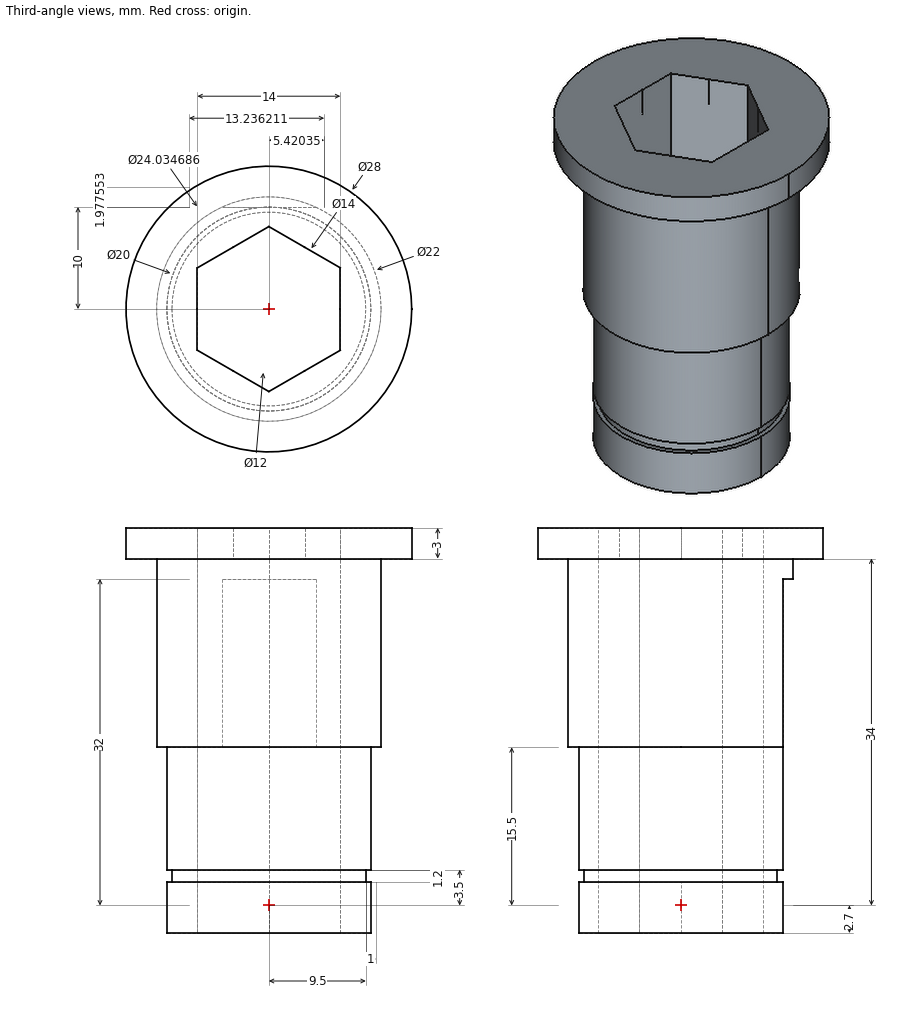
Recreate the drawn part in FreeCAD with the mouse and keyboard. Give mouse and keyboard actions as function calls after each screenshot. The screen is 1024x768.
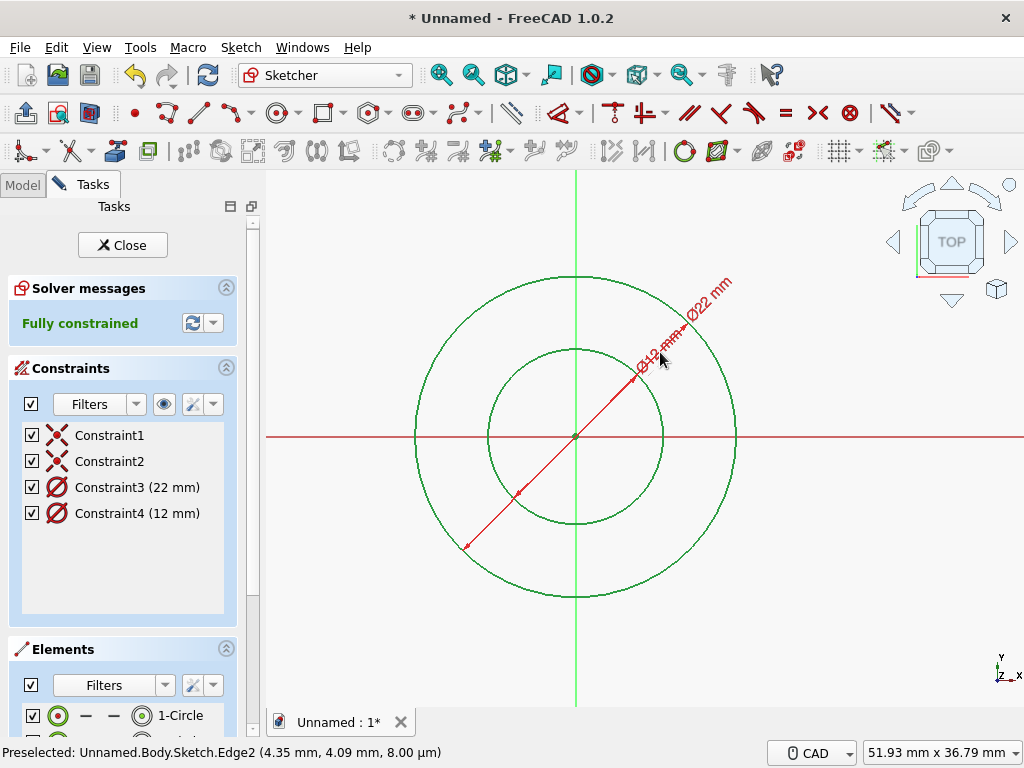
click(123, 245)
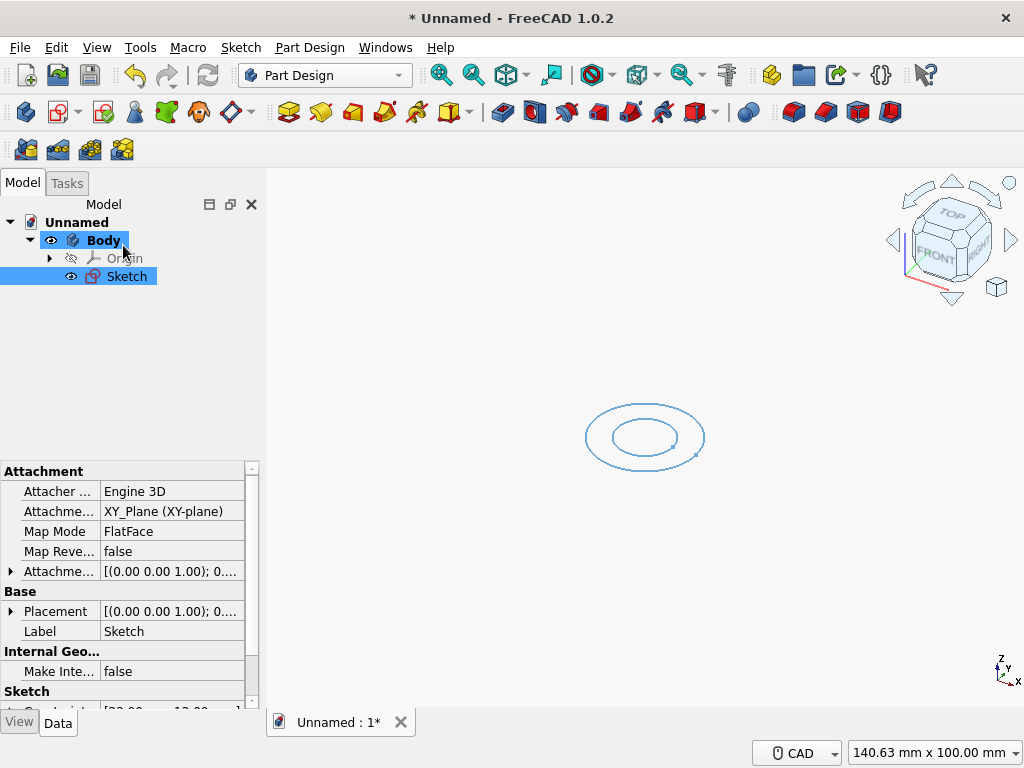
click(290, 112)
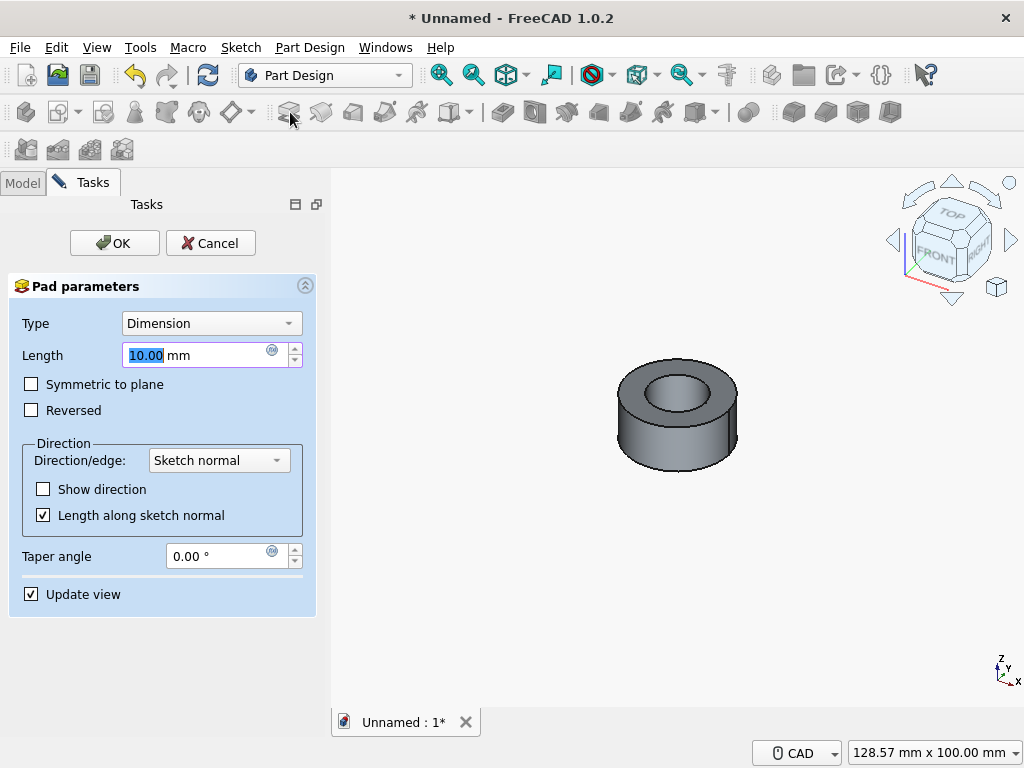
text(34)
key(Tab)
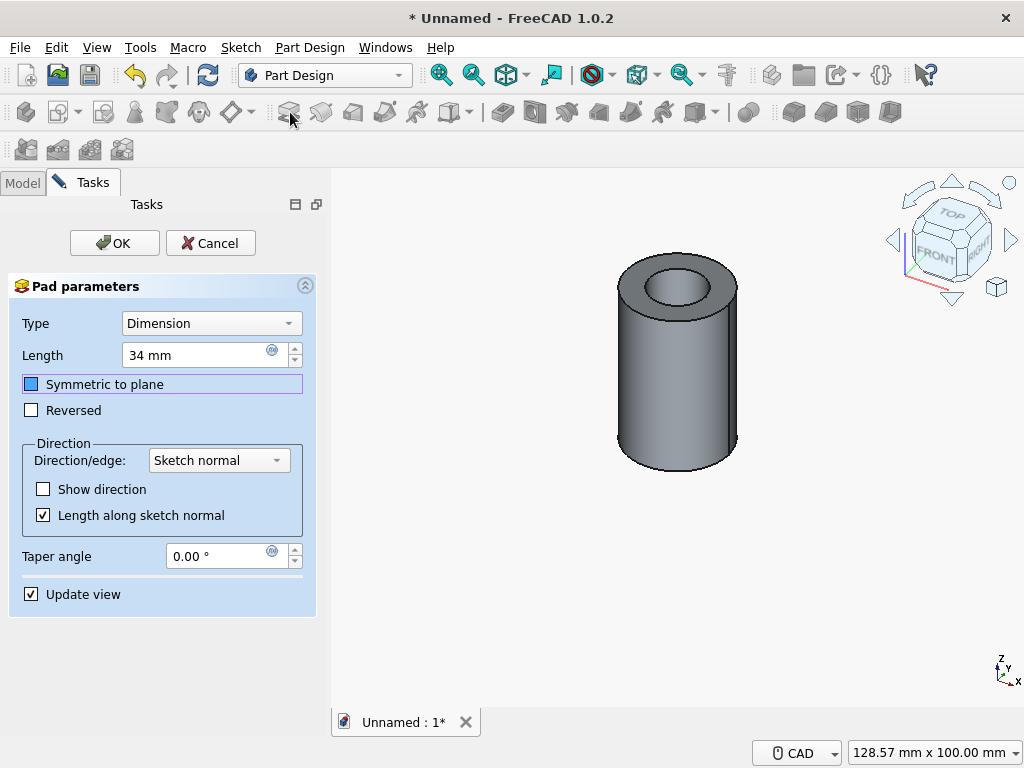
click(115, 243)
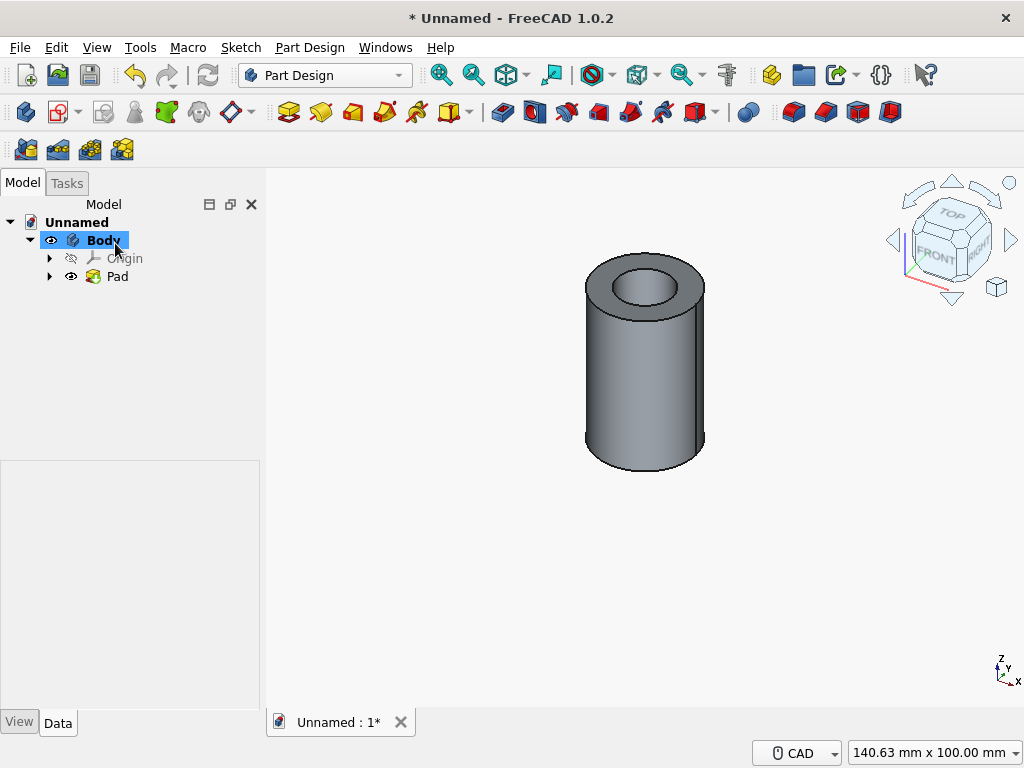
click(691, 279)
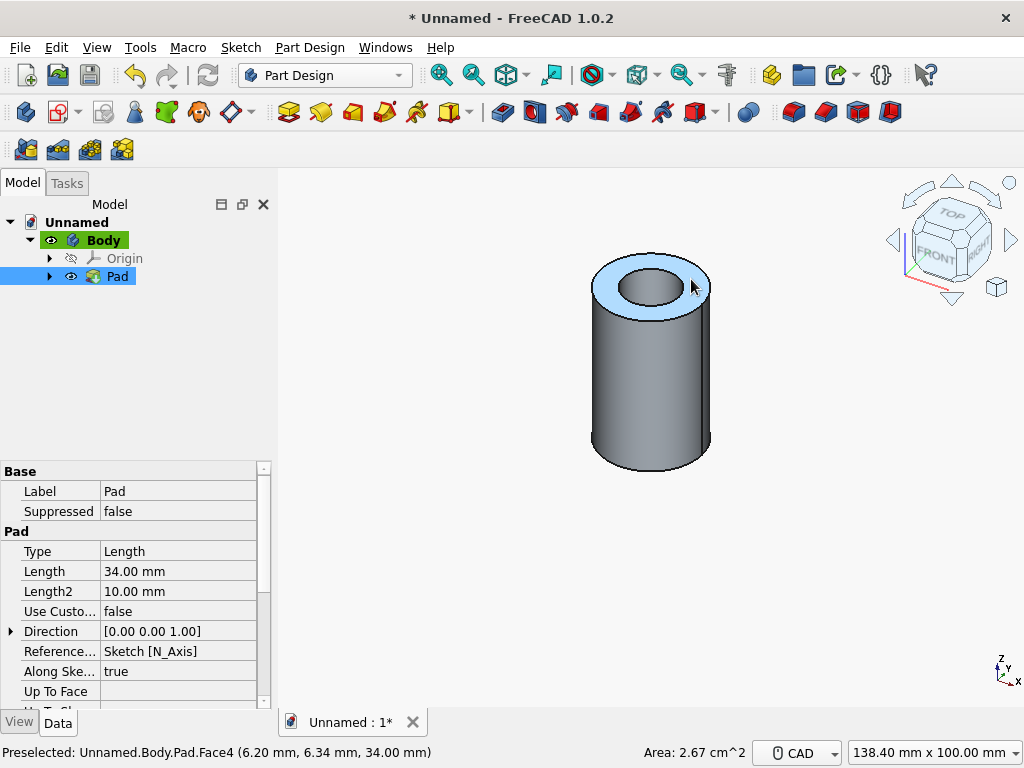
click(58, 112)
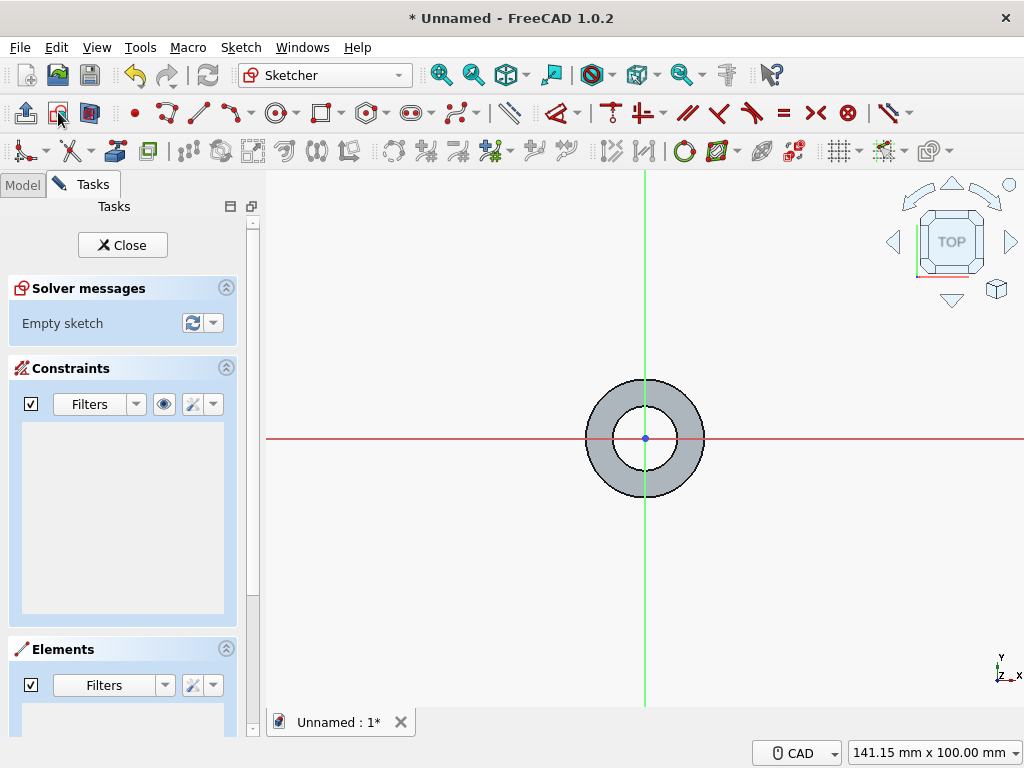
scroll(701, 438, up, 4)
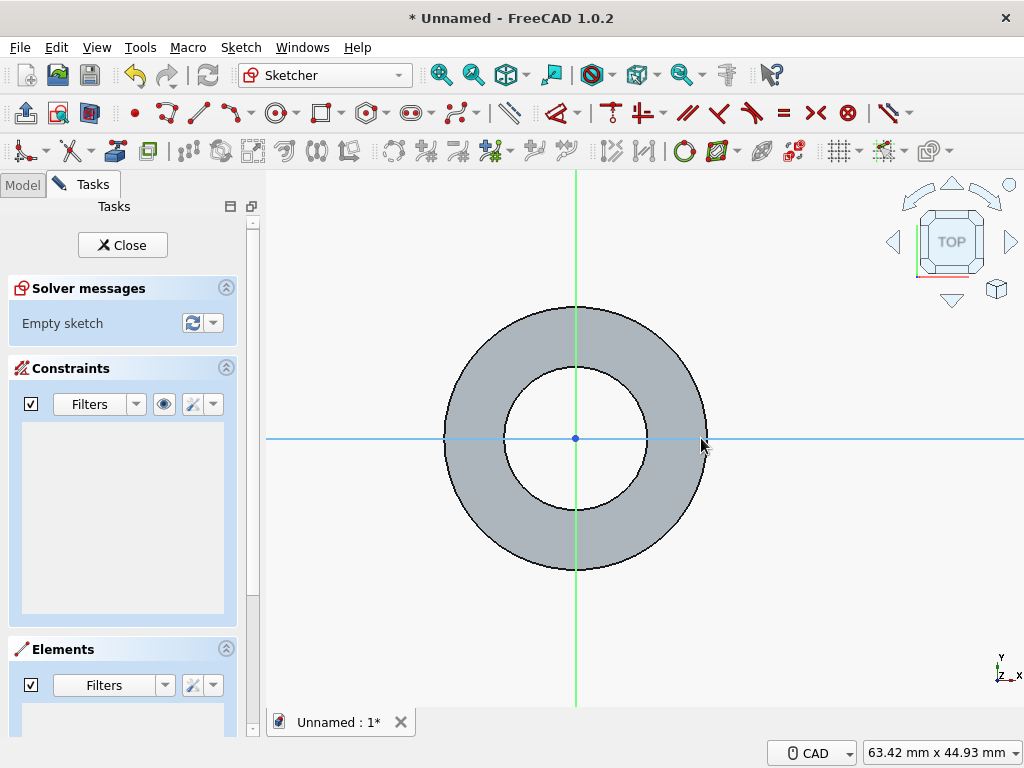
click(276, 114)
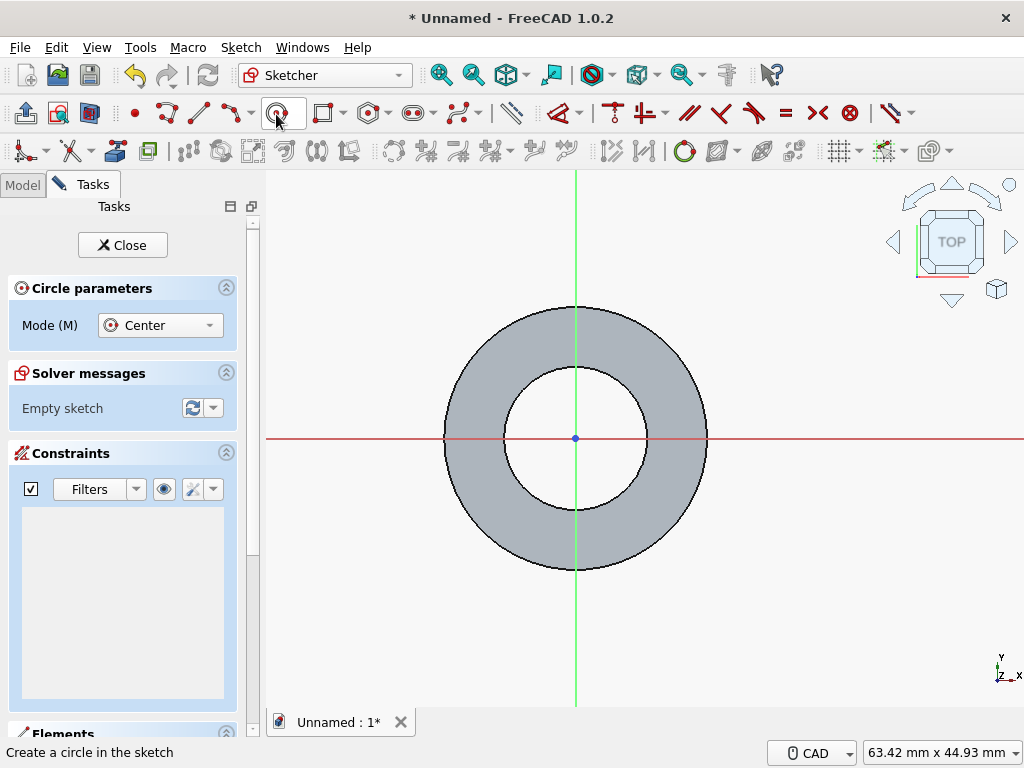
click(576, 438)
click(694, 320)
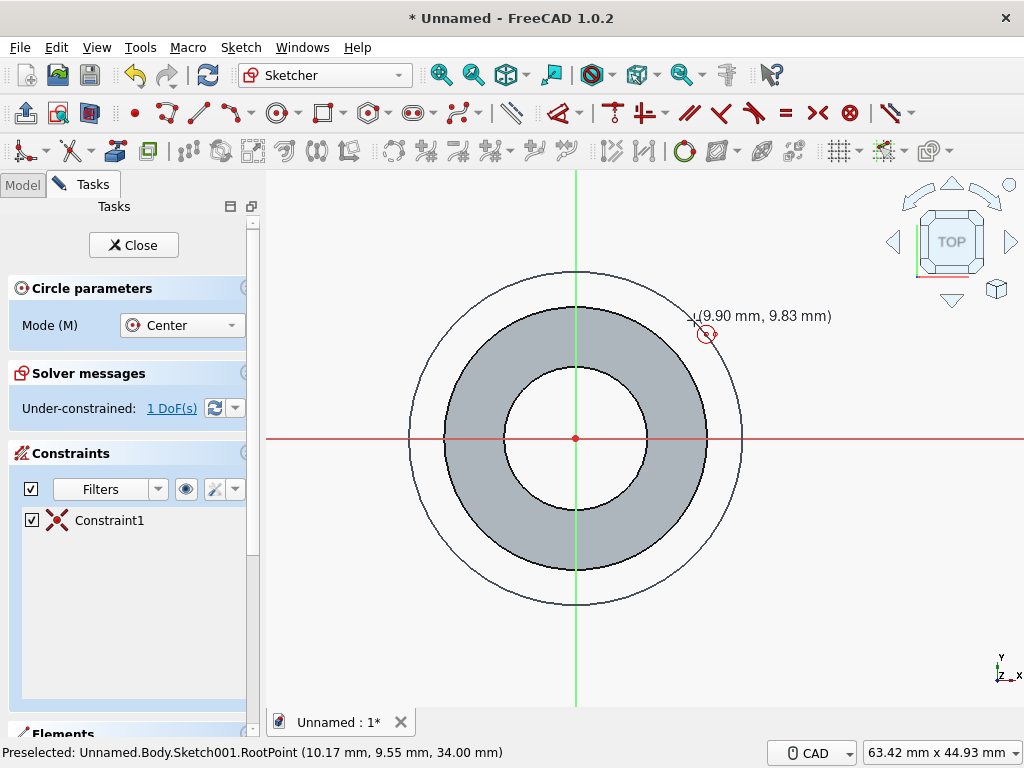
click(576, 438)
click(635, 379)
key(Escape)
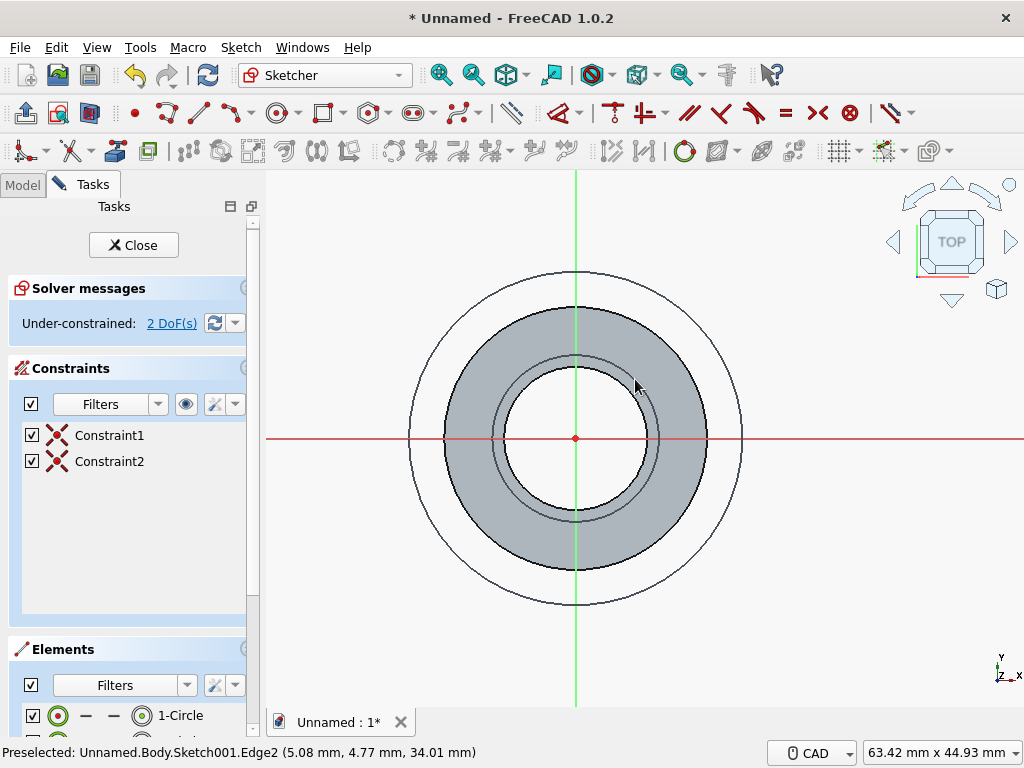
click(558, 114)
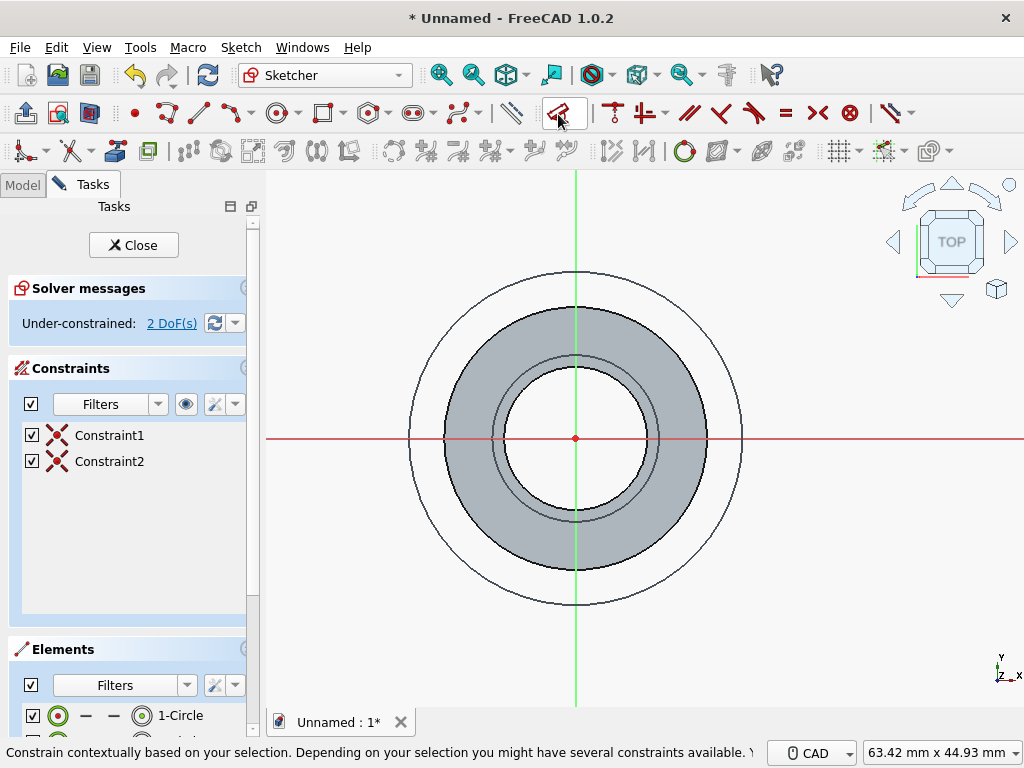
click(693, 320)
click(716, 297)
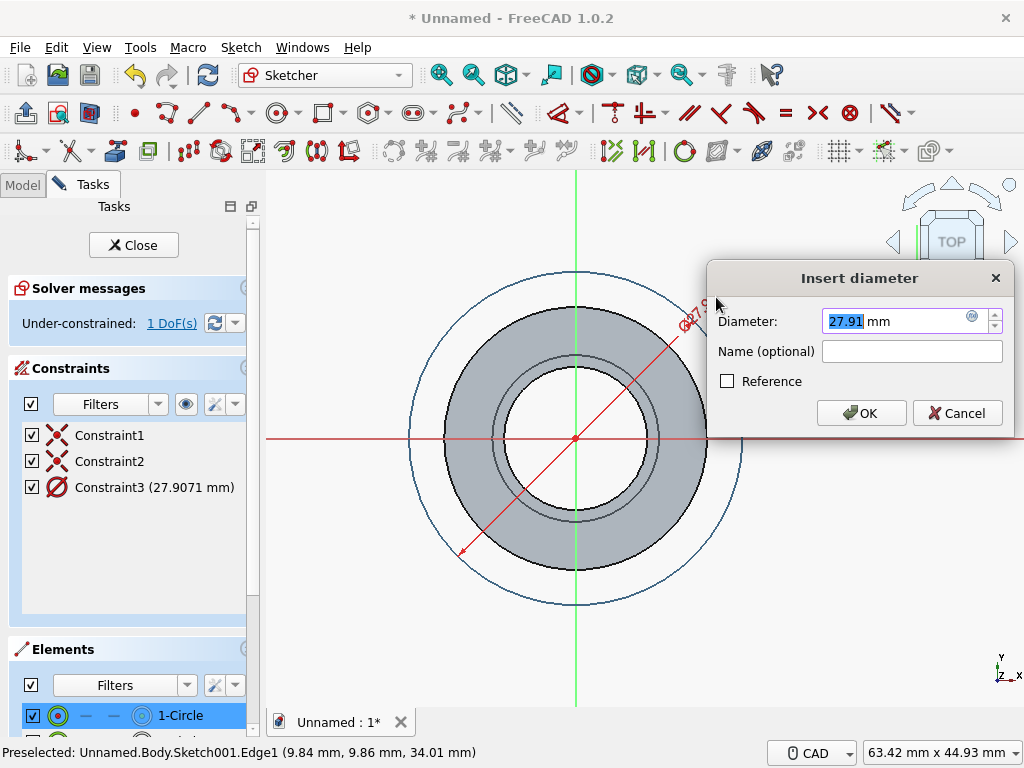
text(28)
key(Return)